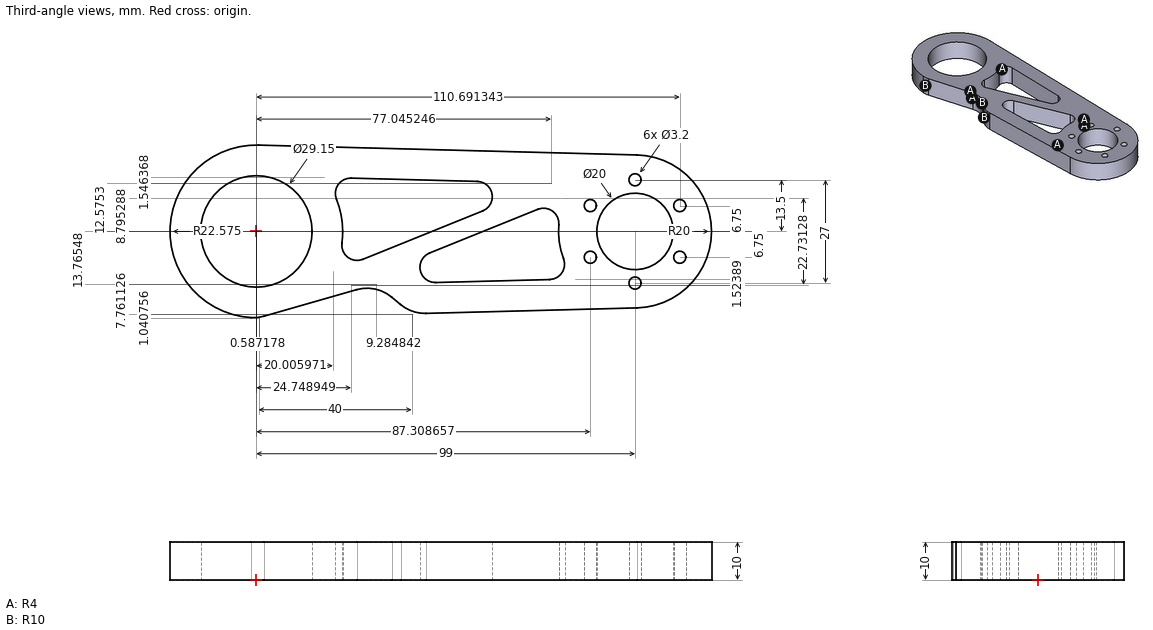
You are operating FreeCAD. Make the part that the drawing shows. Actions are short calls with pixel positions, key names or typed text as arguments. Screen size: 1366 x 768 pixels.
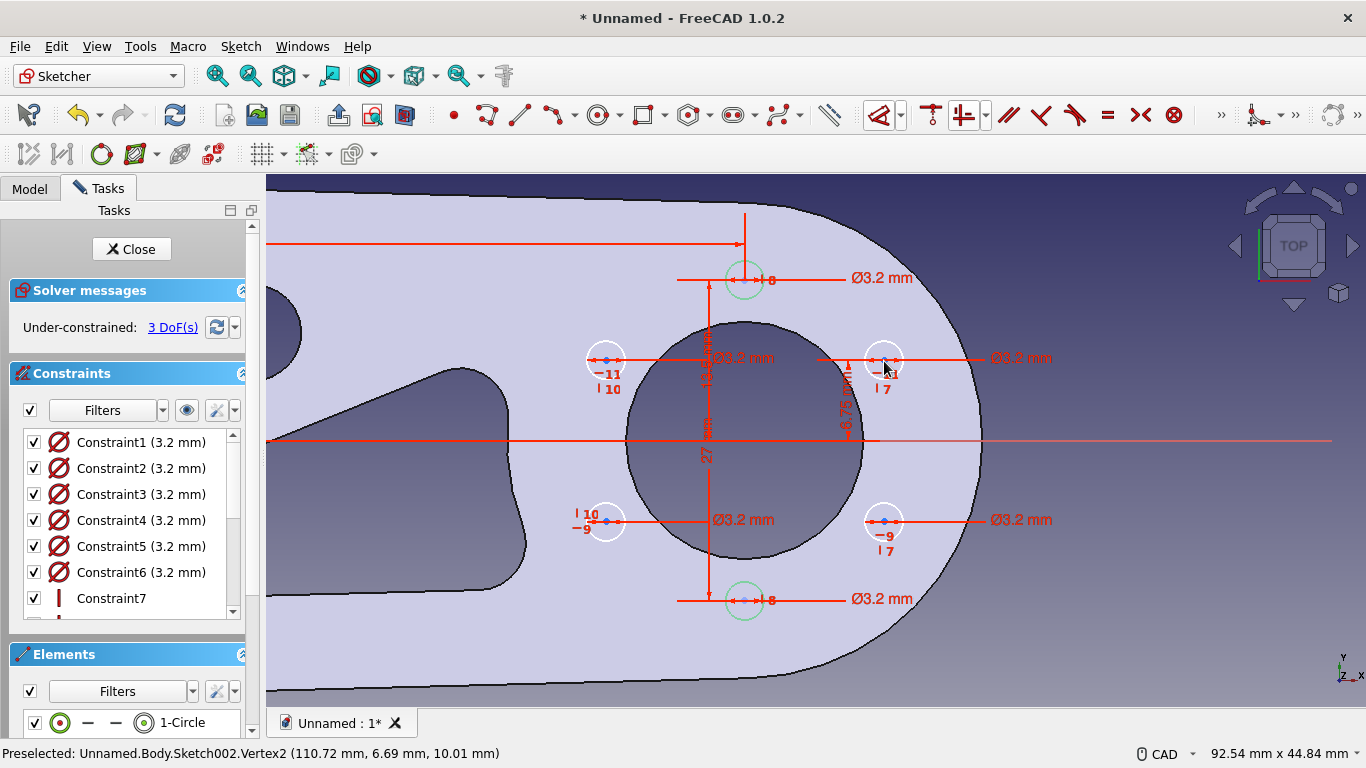
click(884, 522)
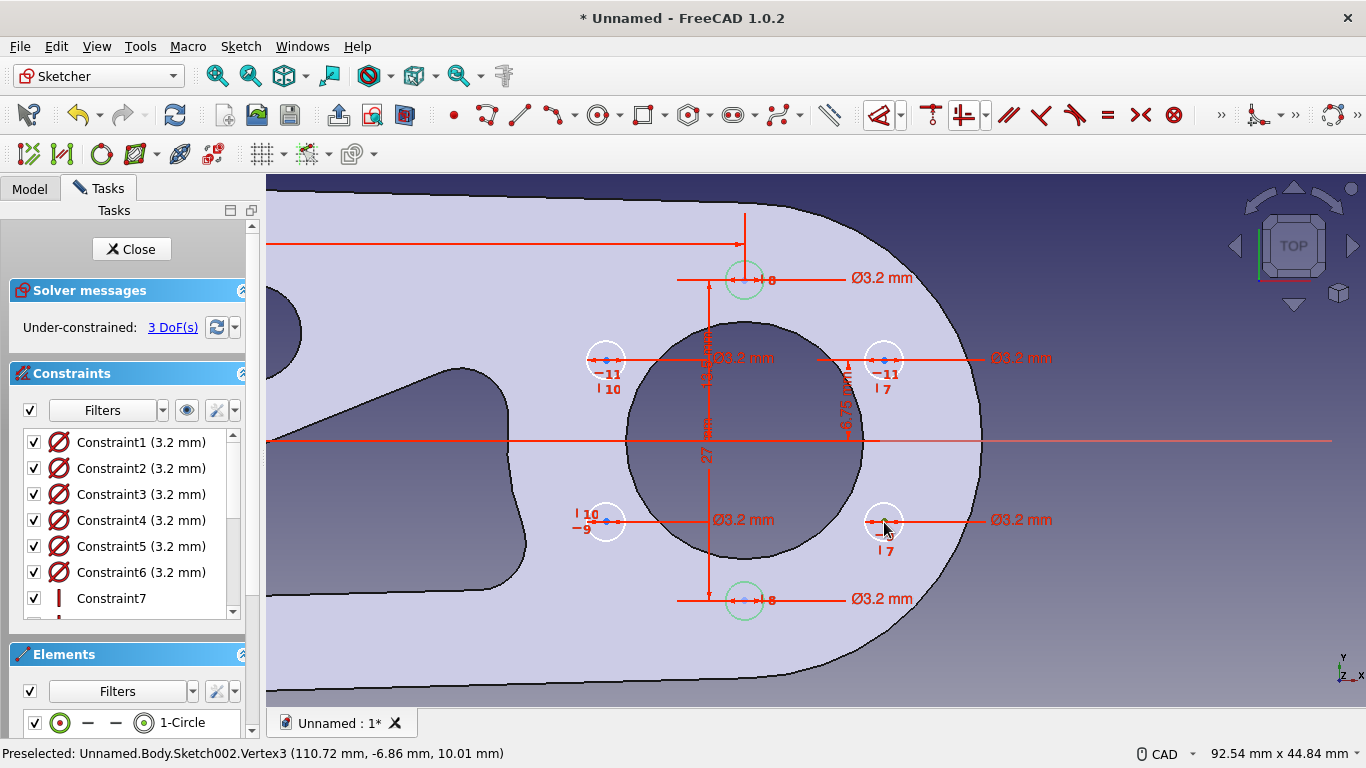
click(900, 116)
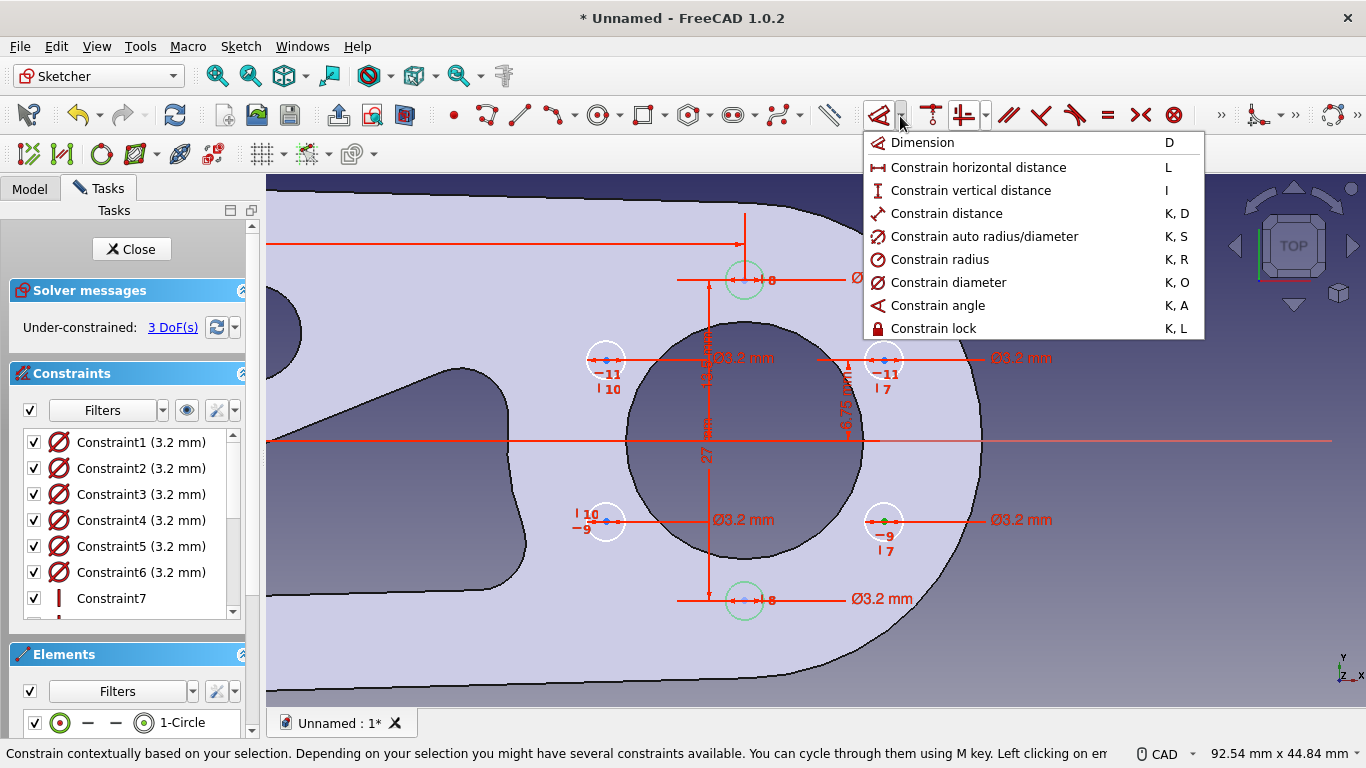
click(1034, 190)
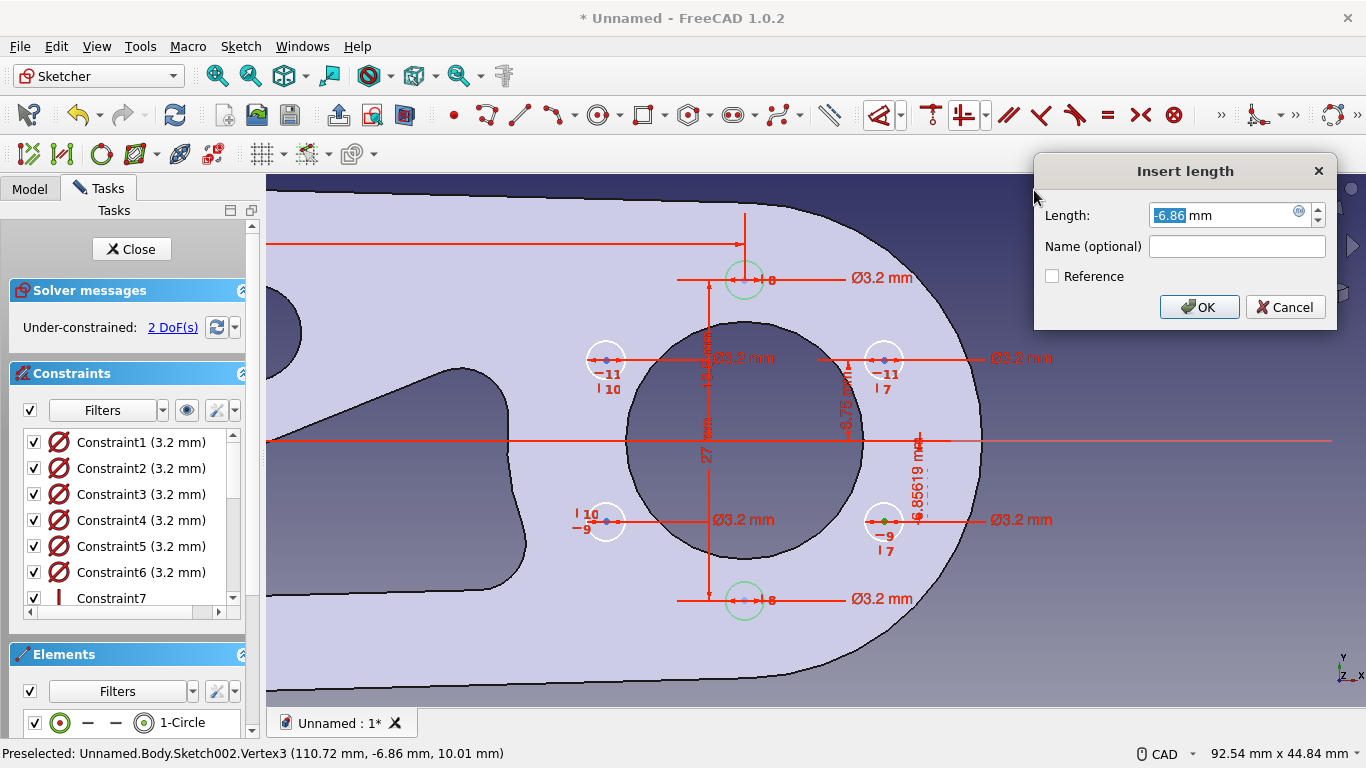
text(-6.75)
key(Return)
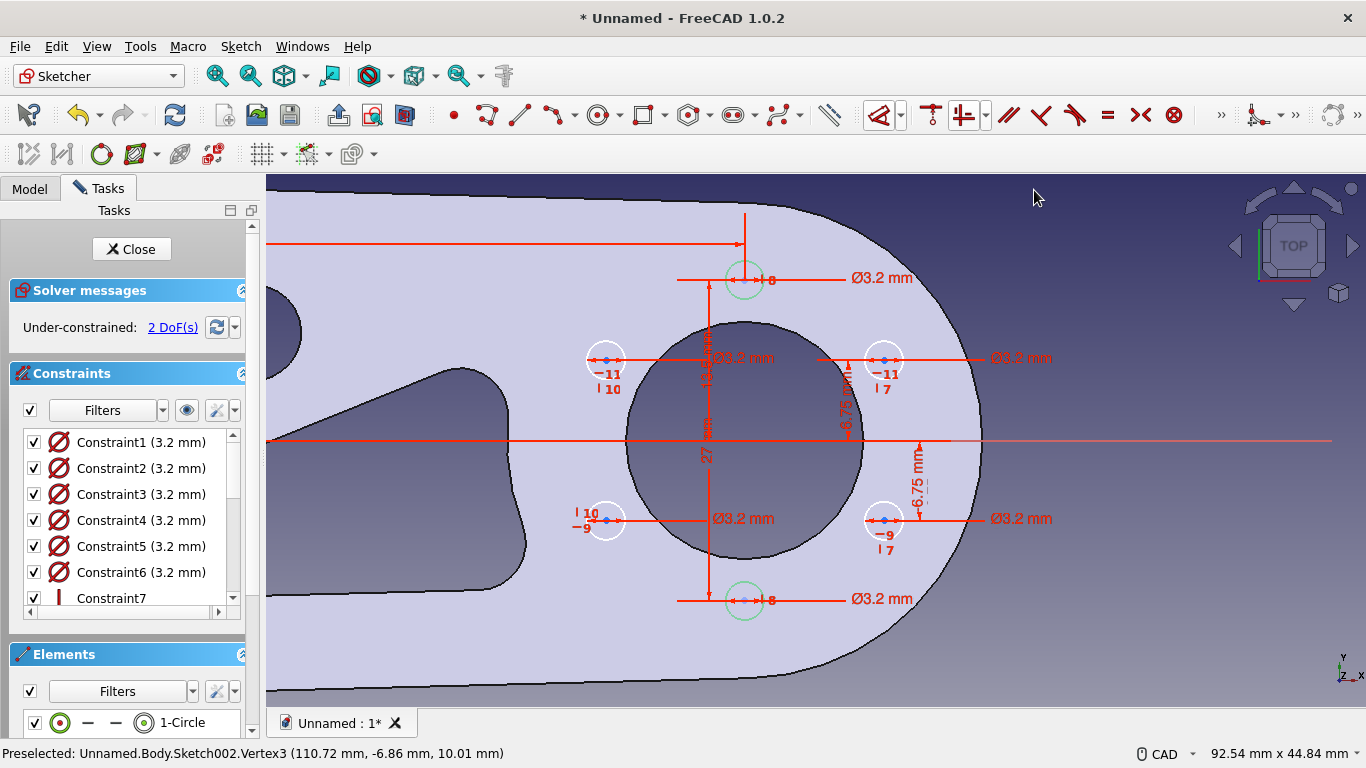
click(606, 521)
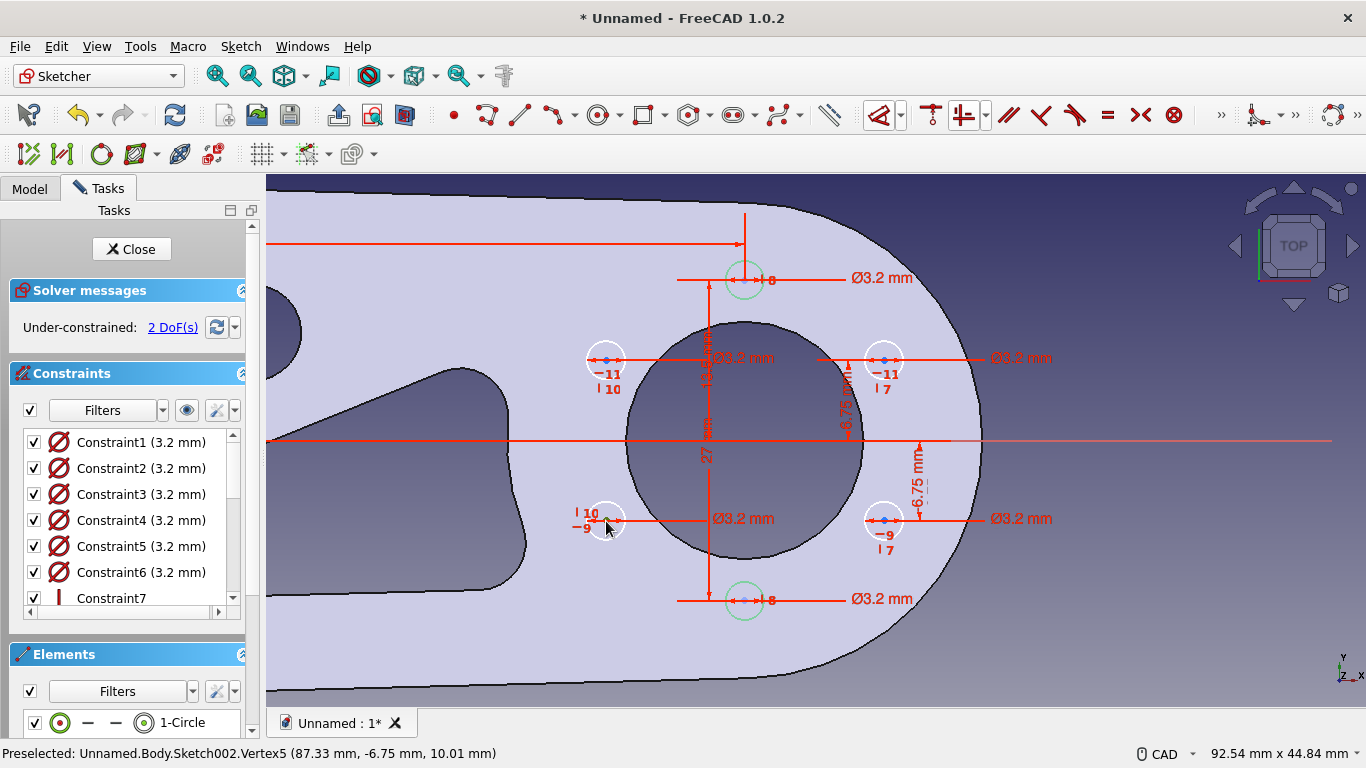
click(900, 116)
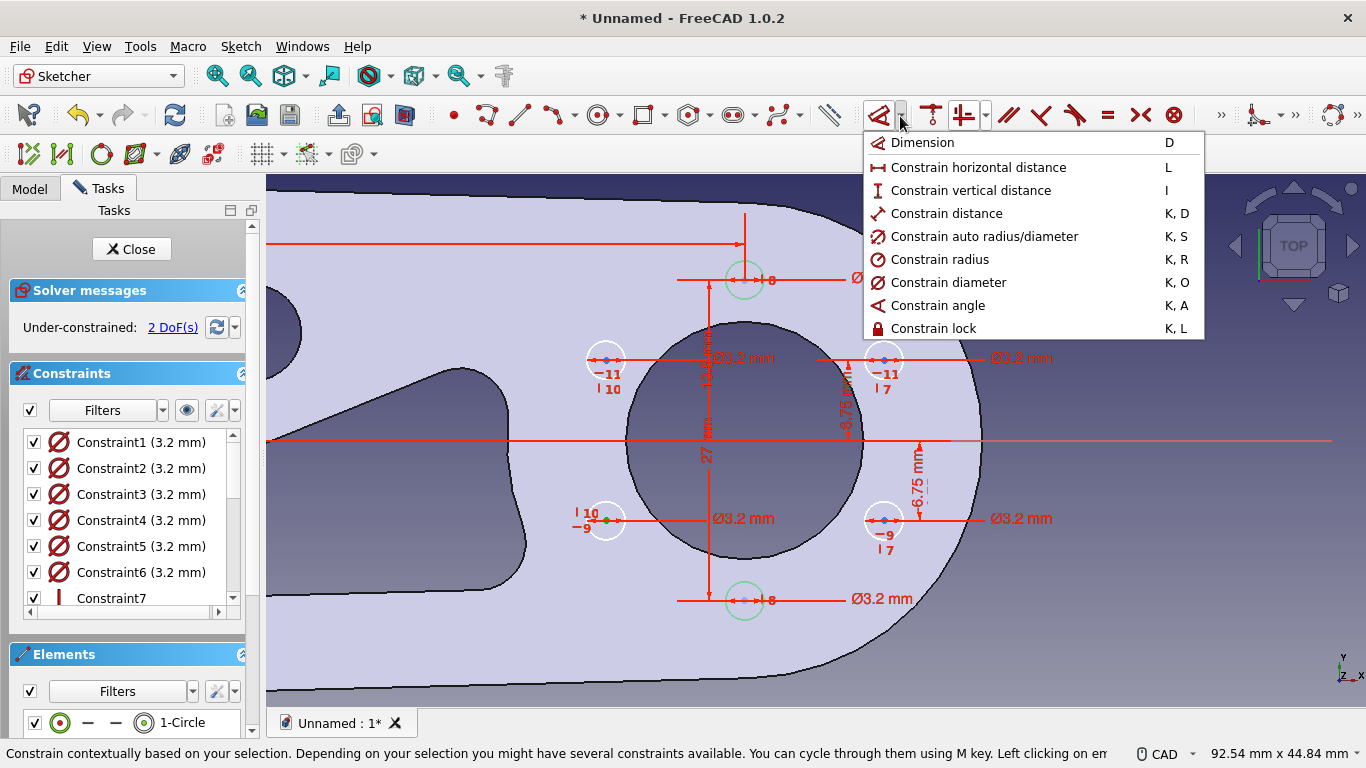
click(1034, 168)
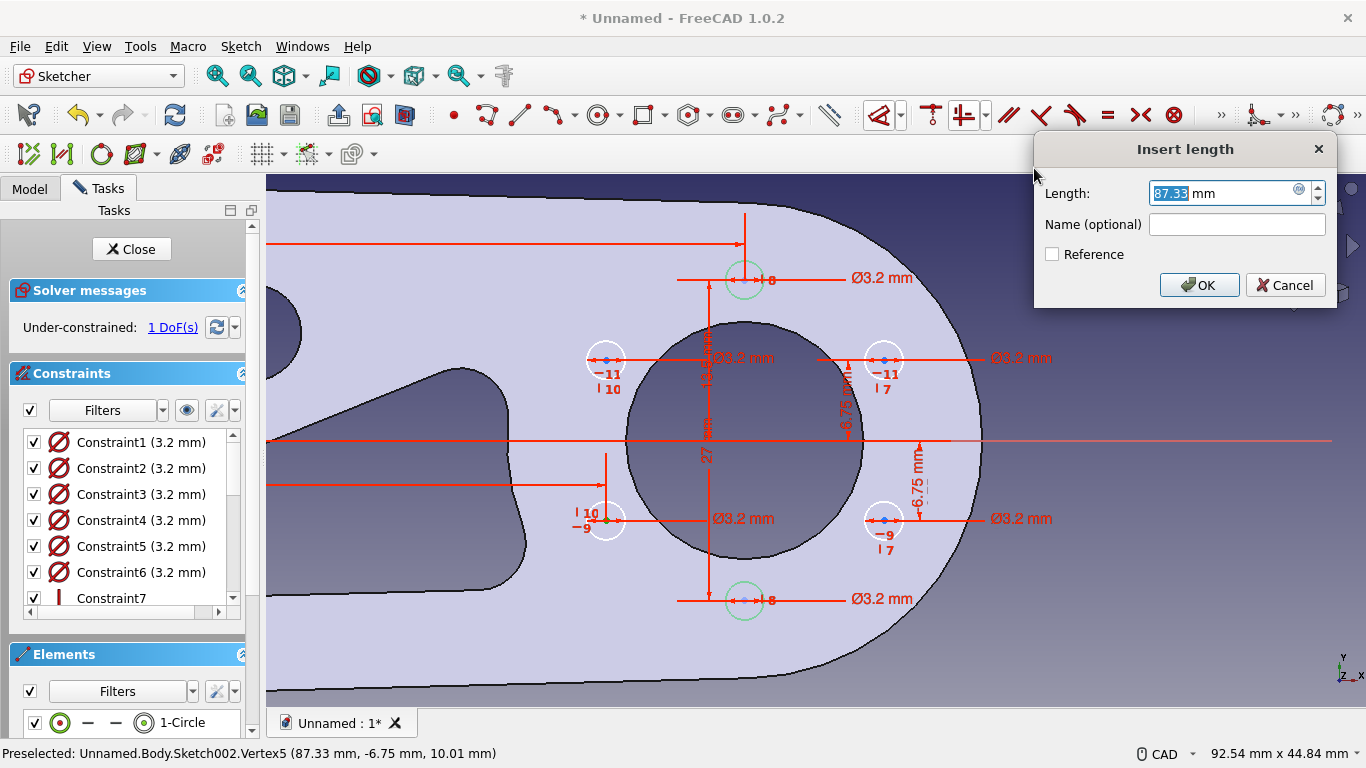
text(87.308657)
key(Return)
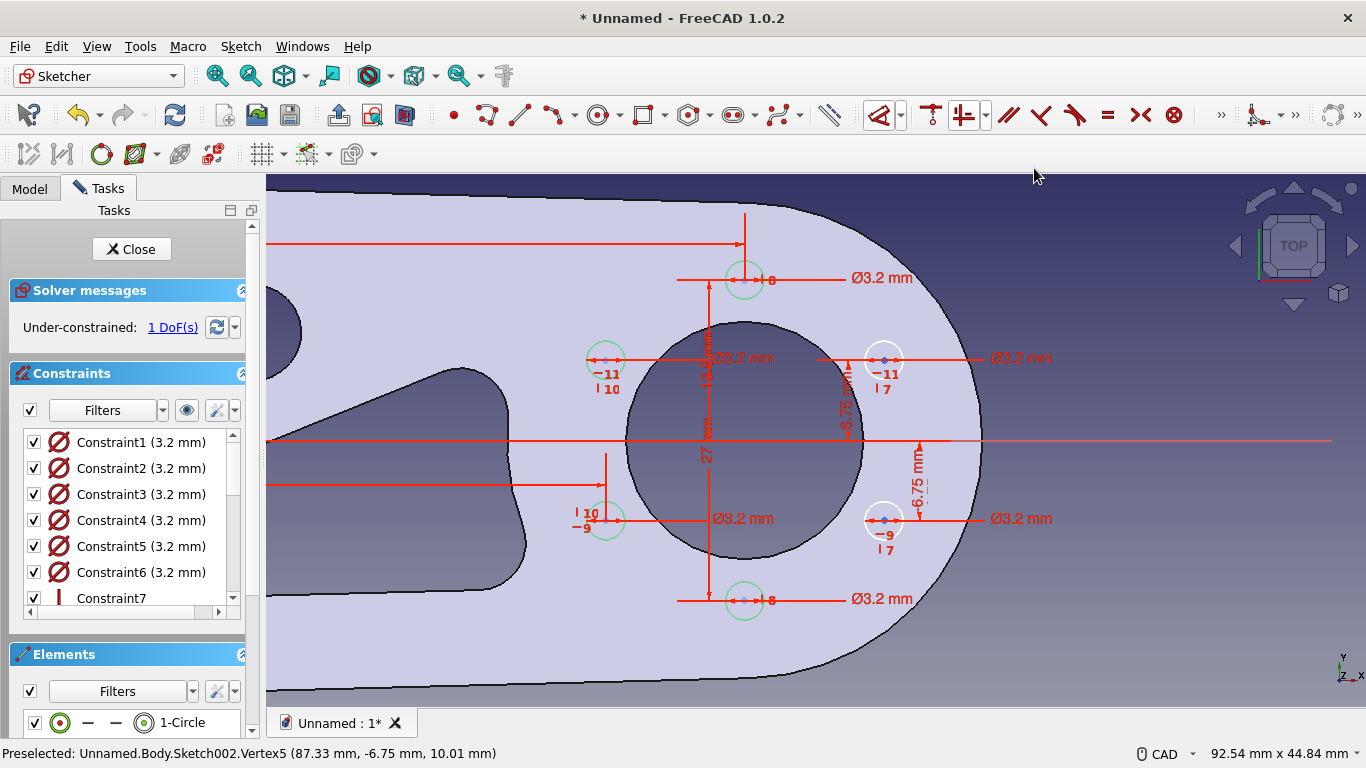
click(884, 360)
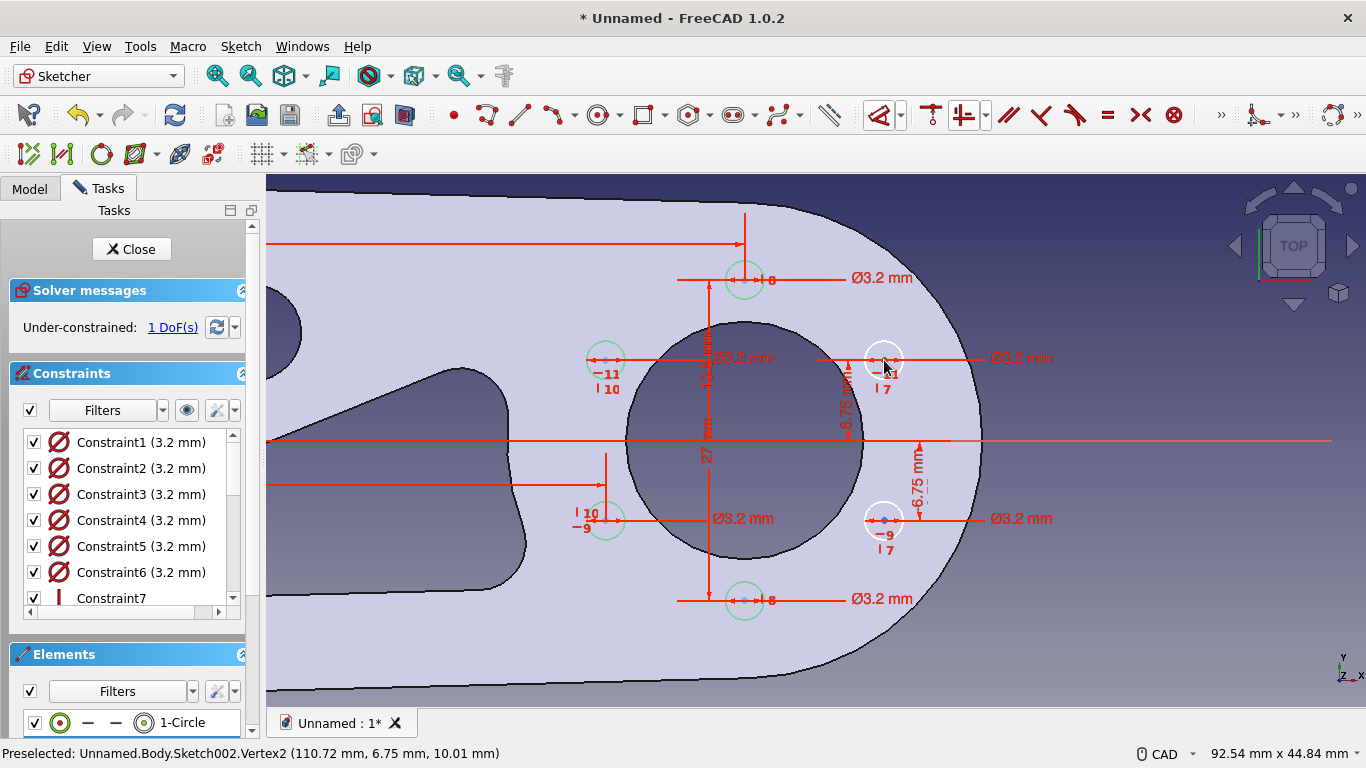
click(900, 116)